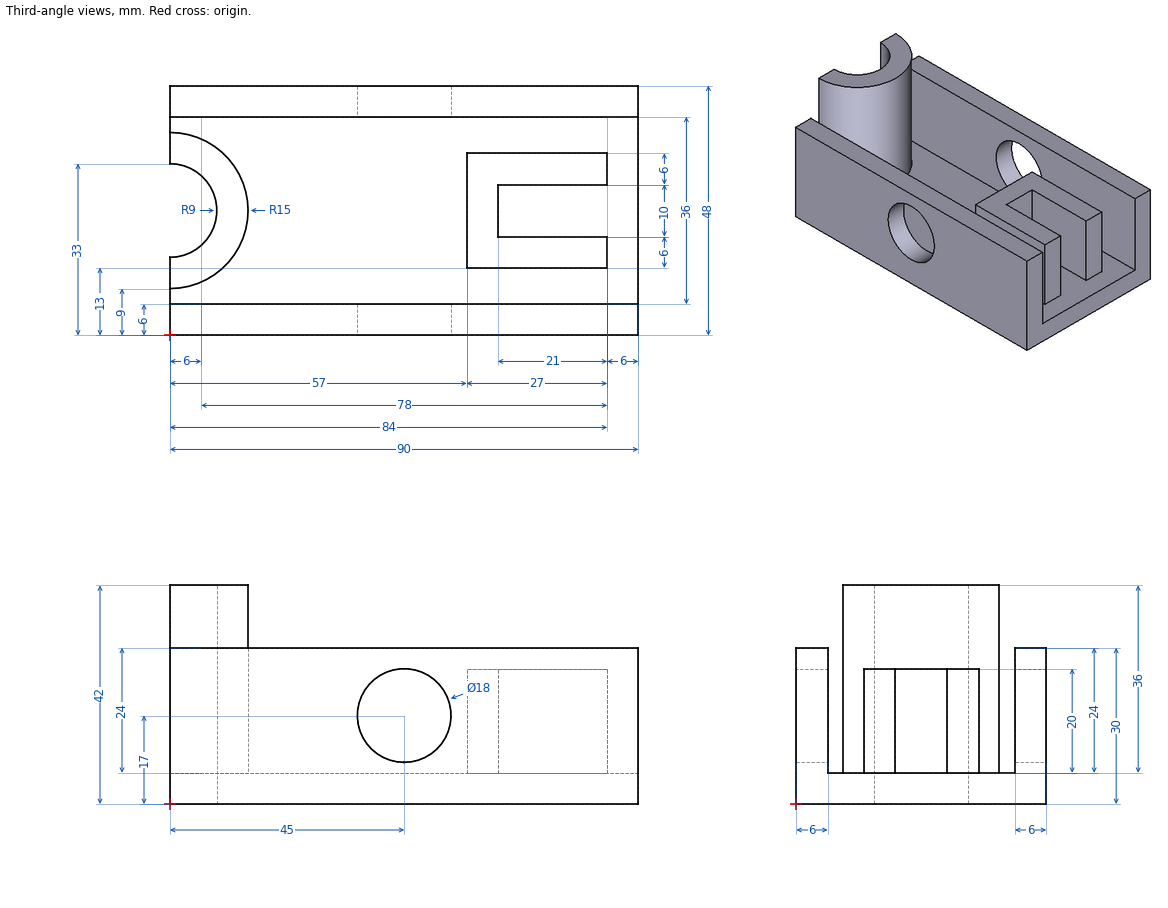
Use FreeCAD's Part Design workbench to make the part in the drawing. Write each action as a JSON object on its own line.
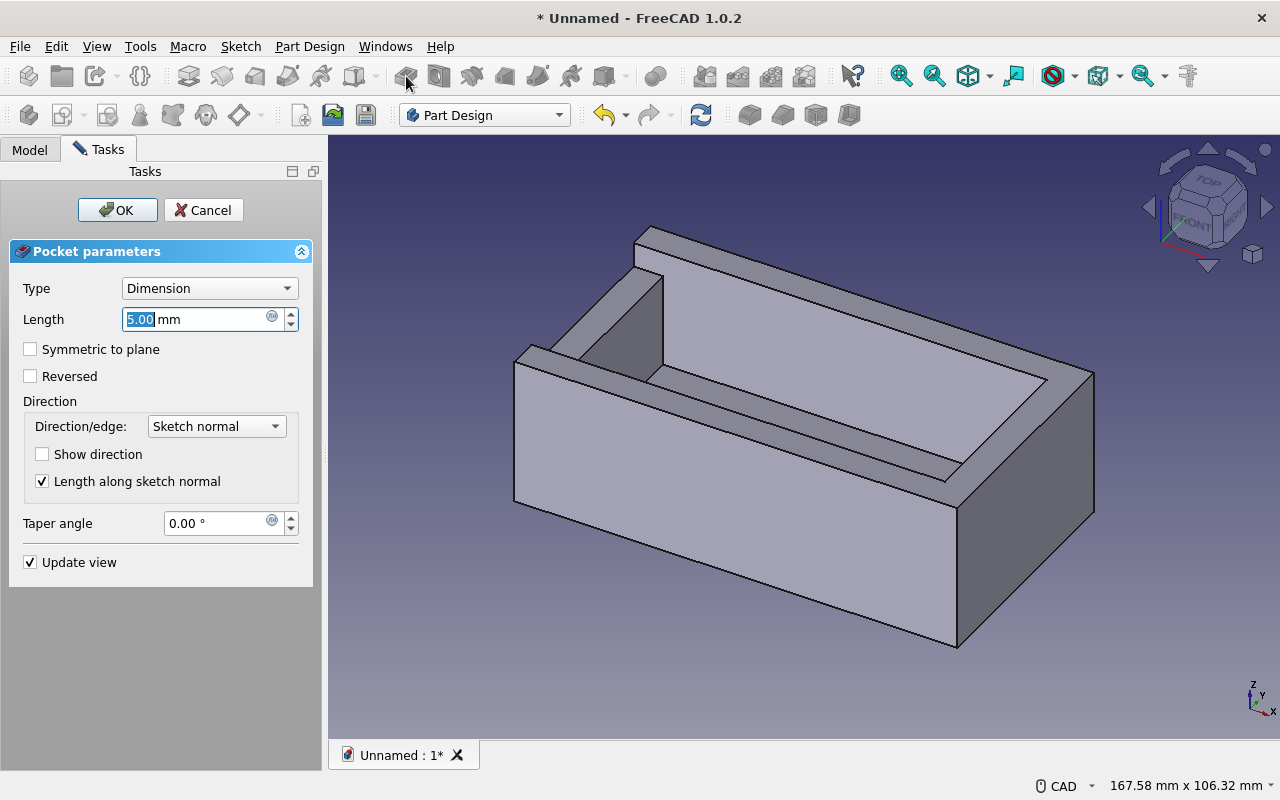
{"action": "type", "text": "24"}
{"action": "key", "text": "Tab"}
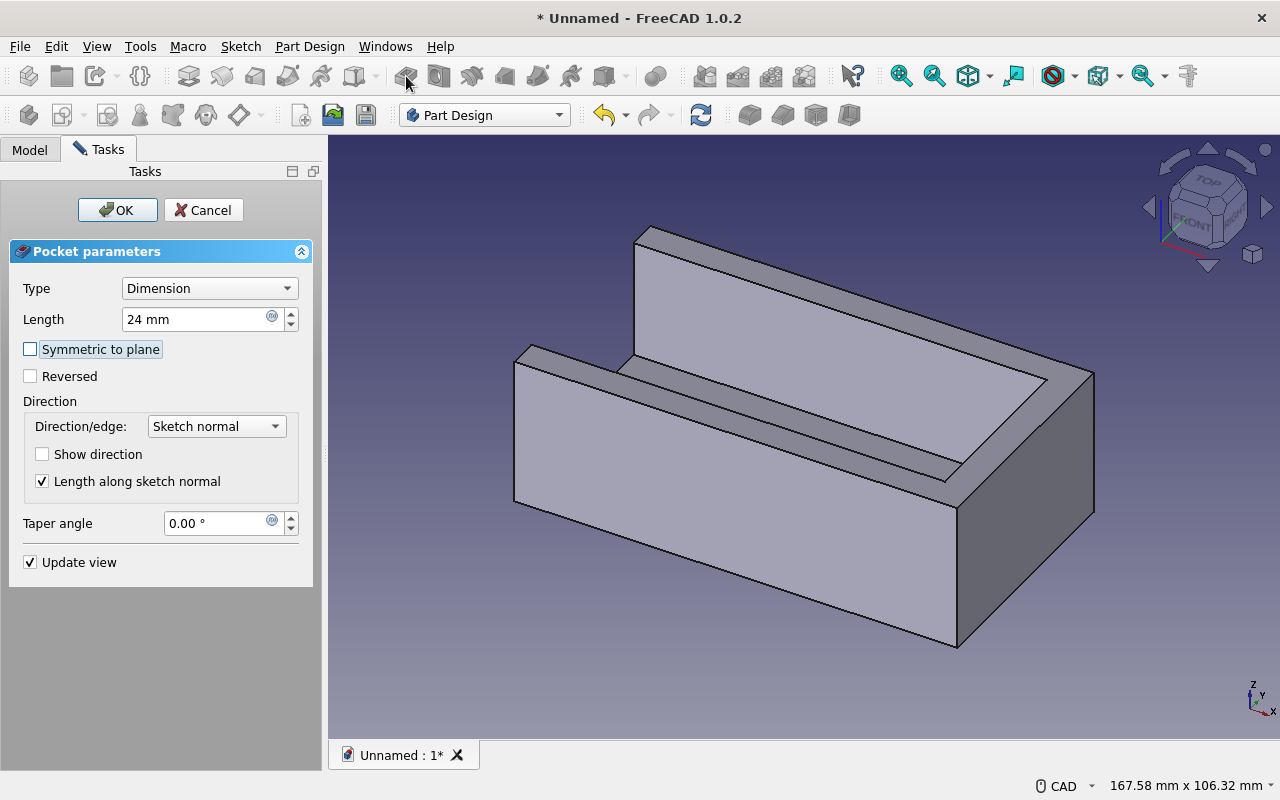
{"action": "left_click", "coordinate": [118, 210]}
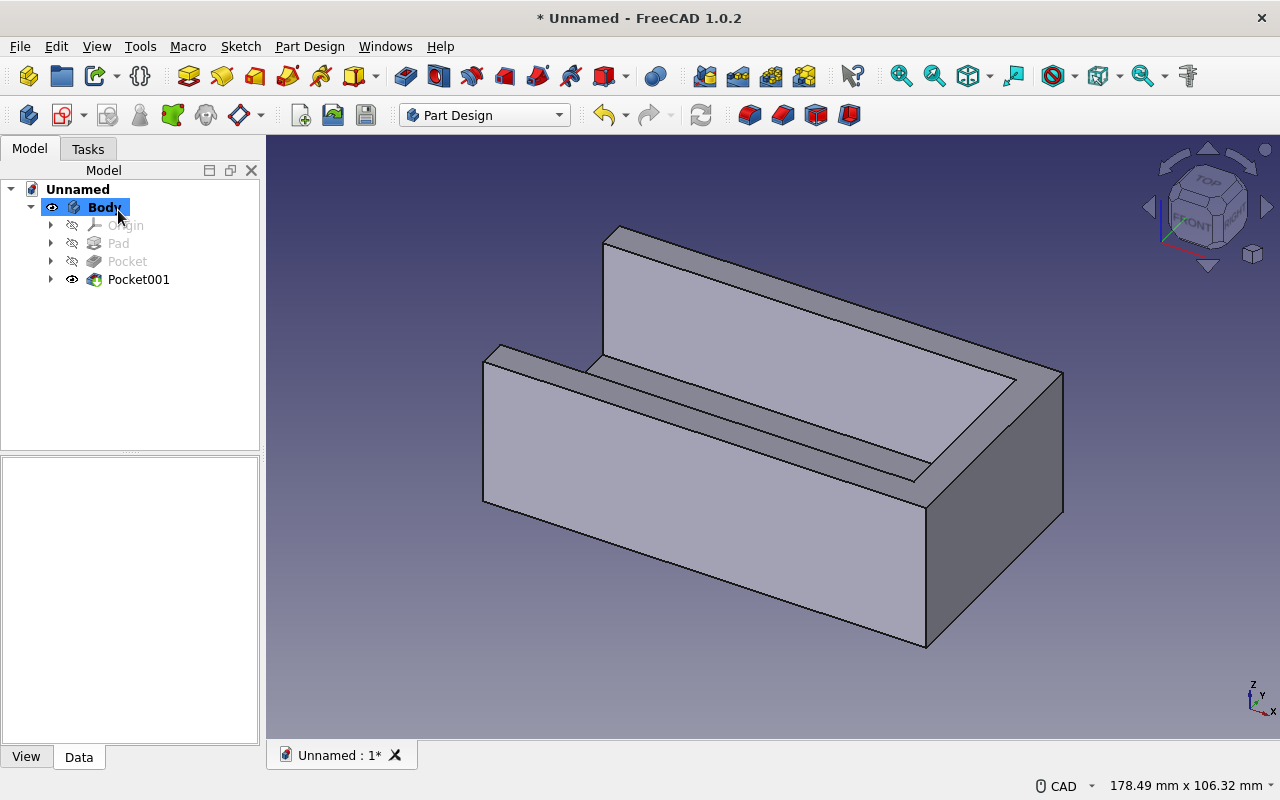
{"action": "left_click", "coordinate": [904, 487]}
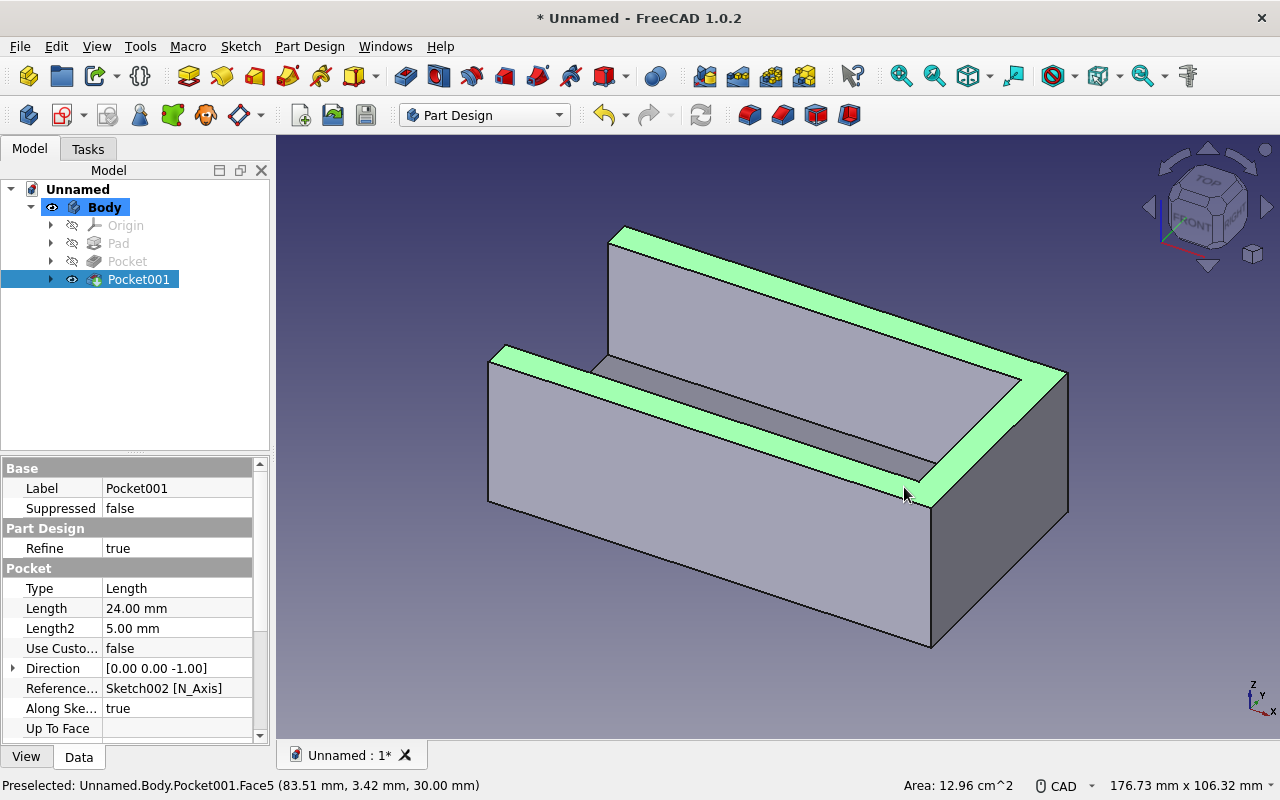
{"action": "left_click", "coordinate": [62, 116]}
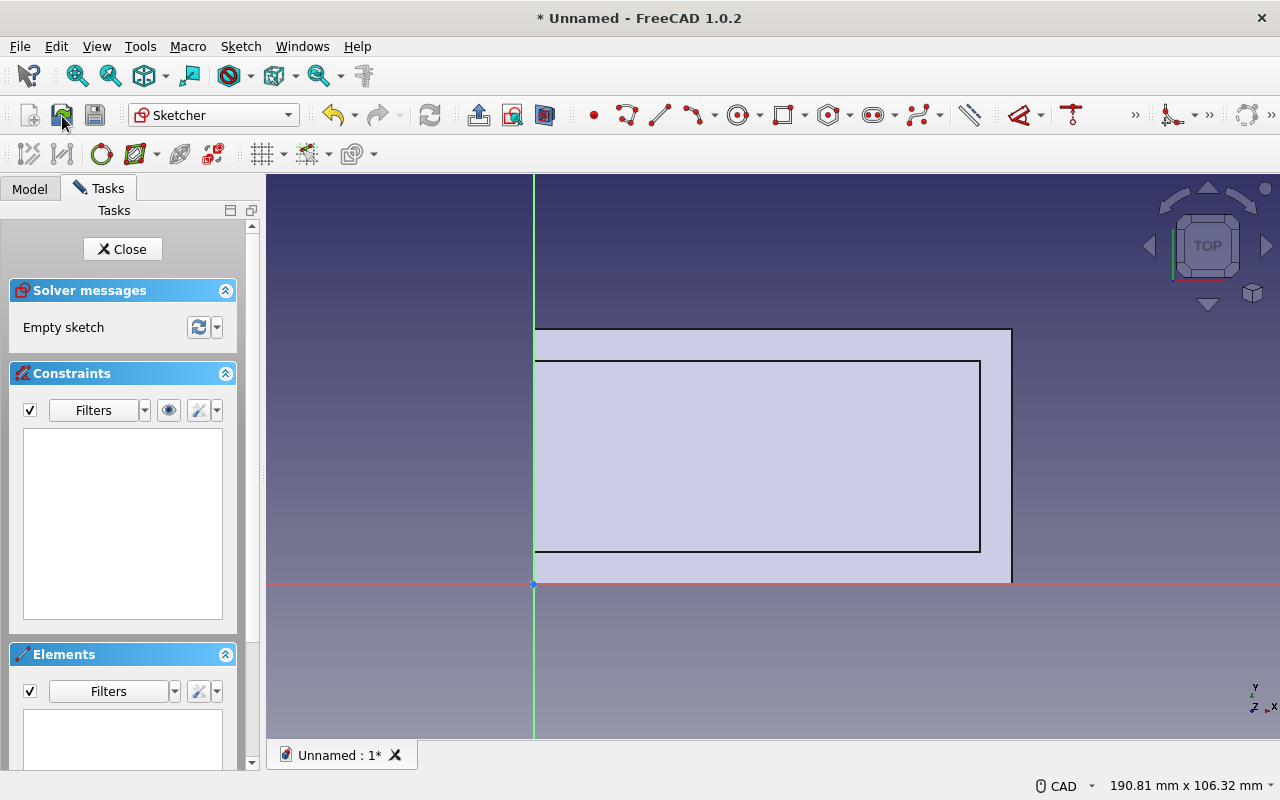
{"action": "scroll", "coordinate": [1115, 456], "scroll_direction": "up", "scroll_amount": 3}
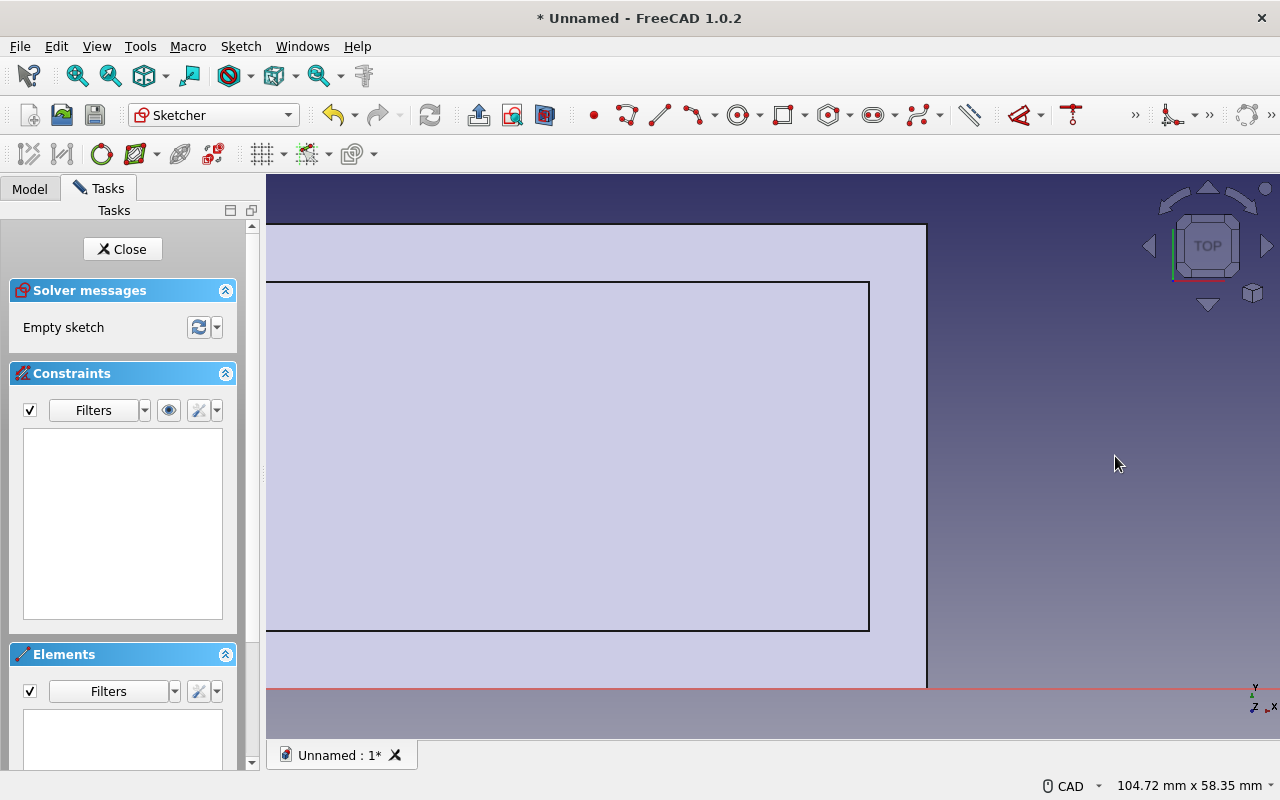
{"action": "key", "text": "g r"}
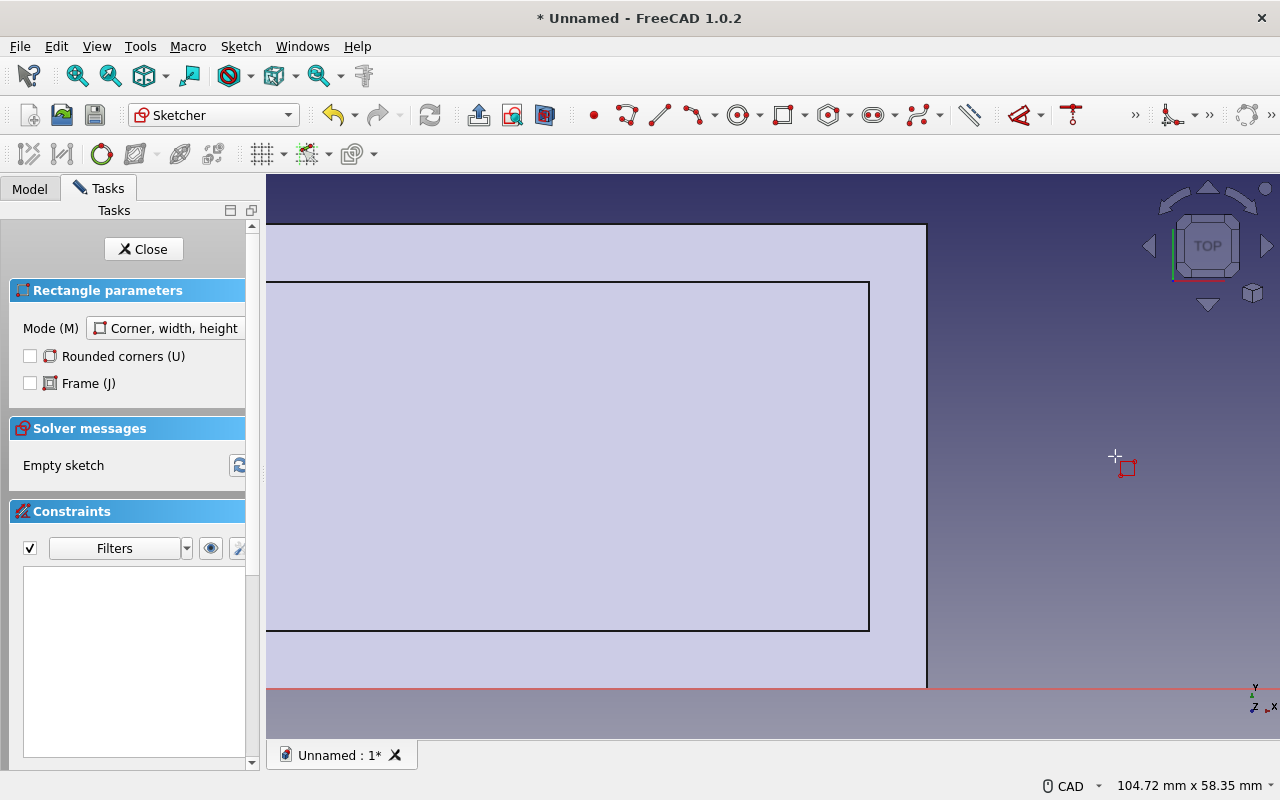
{"action": "left_click", "coordinate": [869, 282]}
{"action": "mouse_move", "coordinate": [927, 631]}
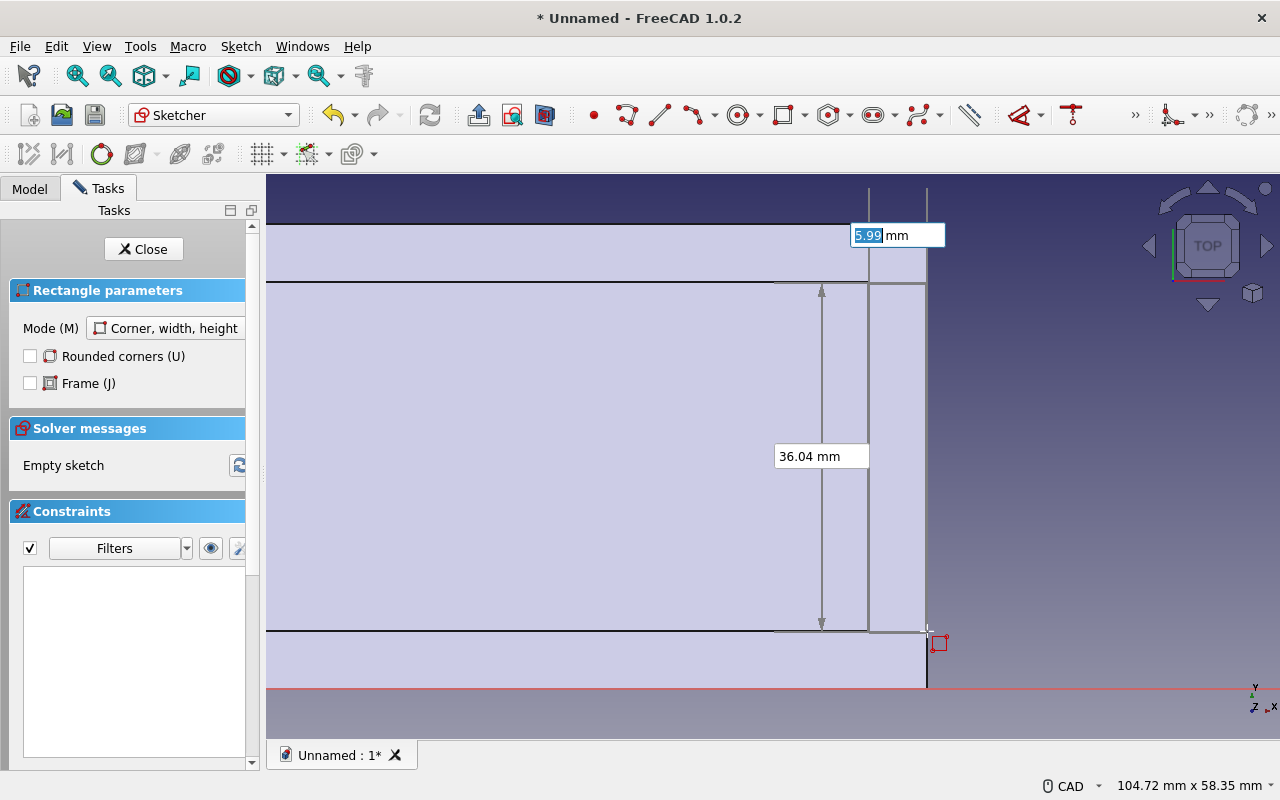
{"action": "type", "text": "6"}
{"action": "key", "text": "Tab"}
{"action": "type", "text": "36"}
{"action": "key", "text": "Return"}
{"action": "key", "text": "Escape"}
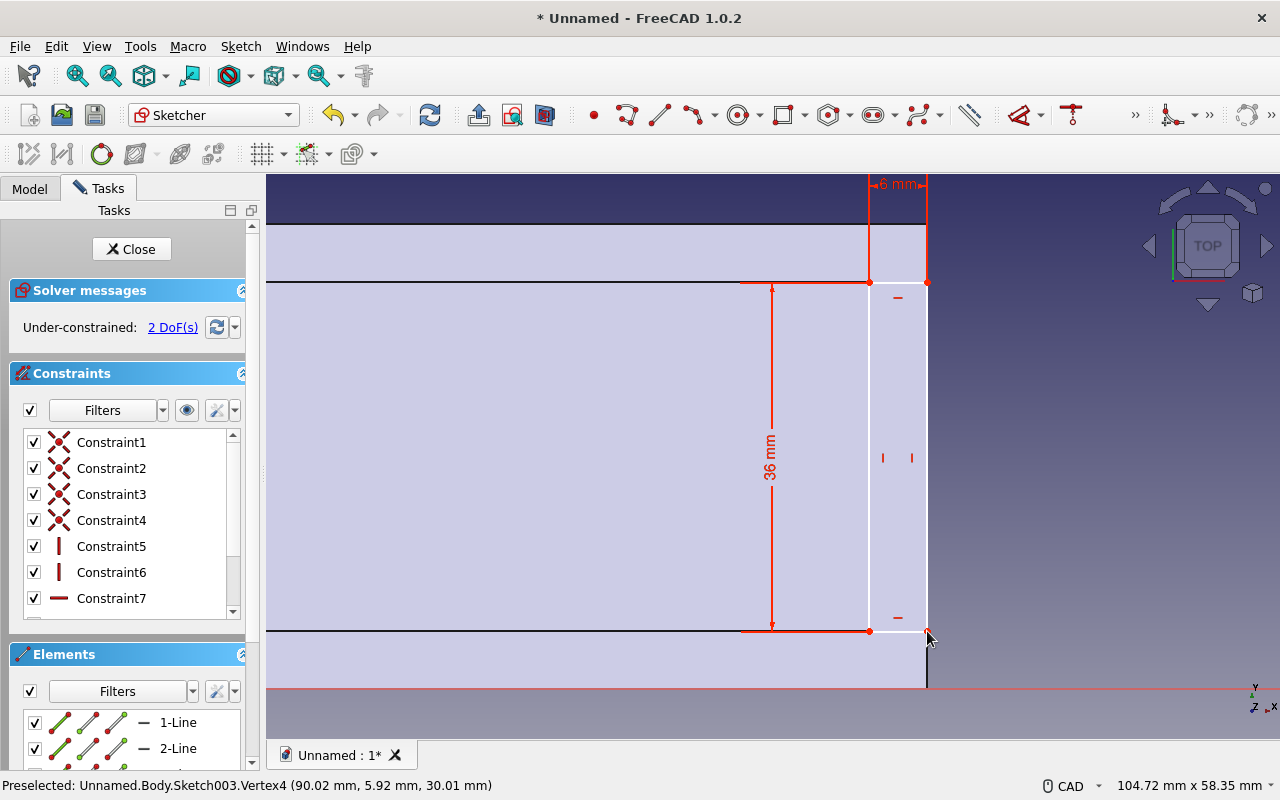
{"action": "key", "text": "d"}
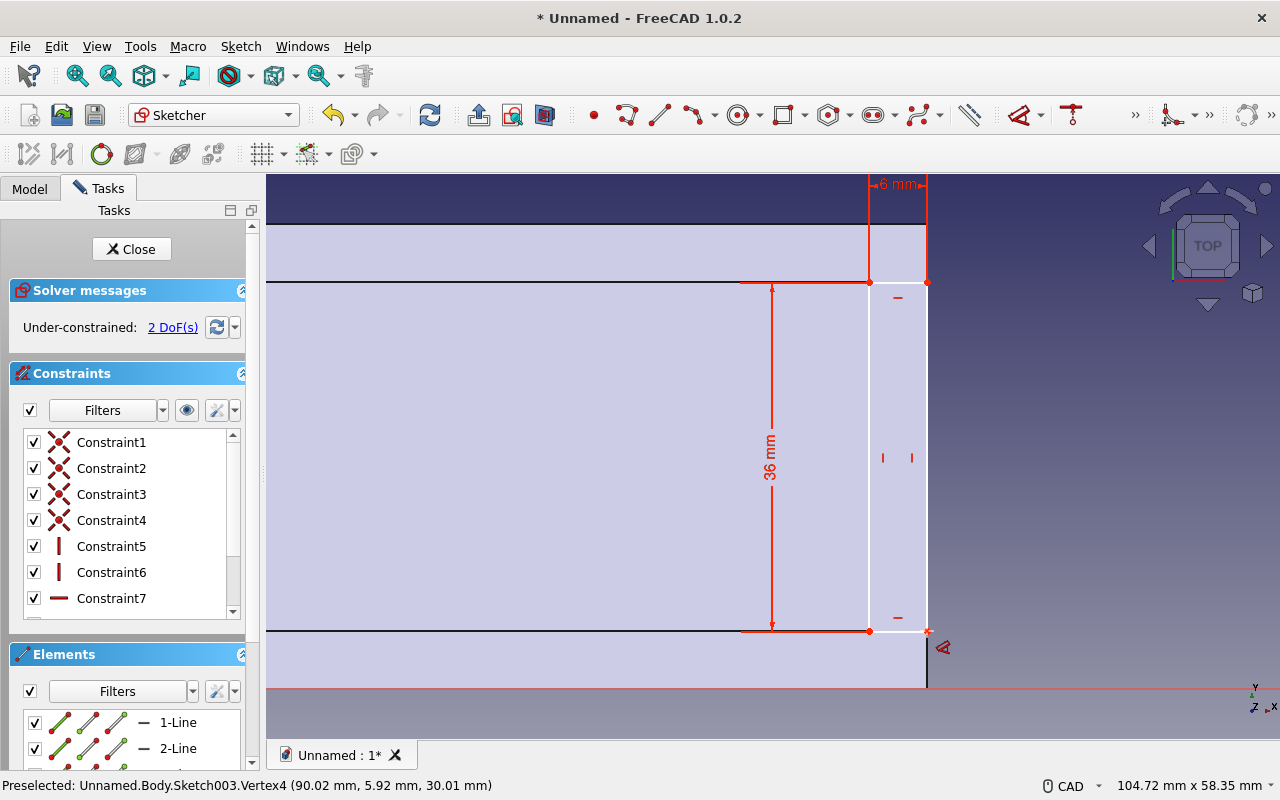
{"action": "left_click", "coordinate": [869, 632]}
{"action": "left_click", "coordinate": [903, 660]}